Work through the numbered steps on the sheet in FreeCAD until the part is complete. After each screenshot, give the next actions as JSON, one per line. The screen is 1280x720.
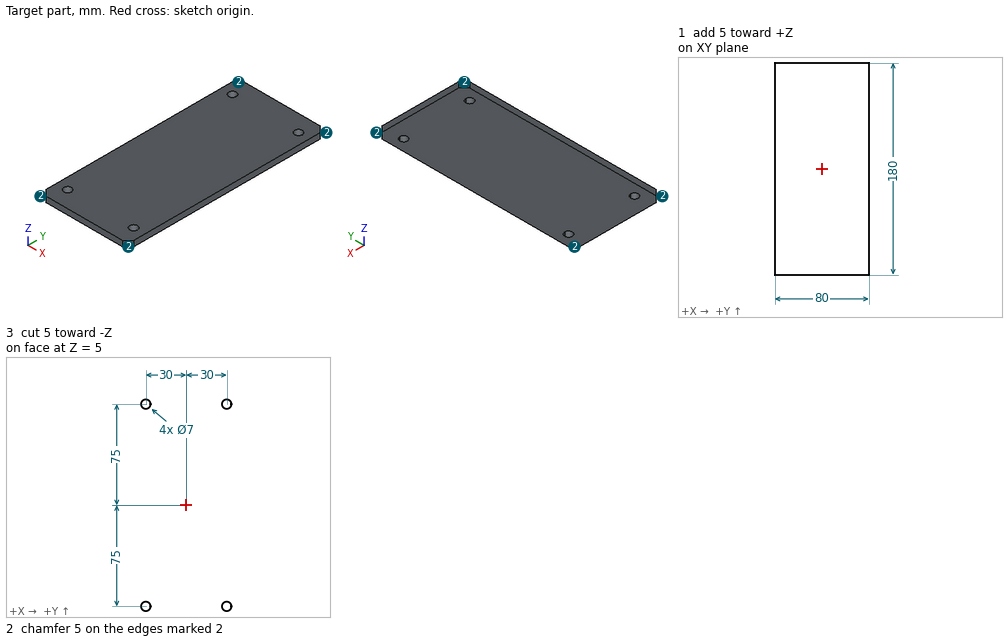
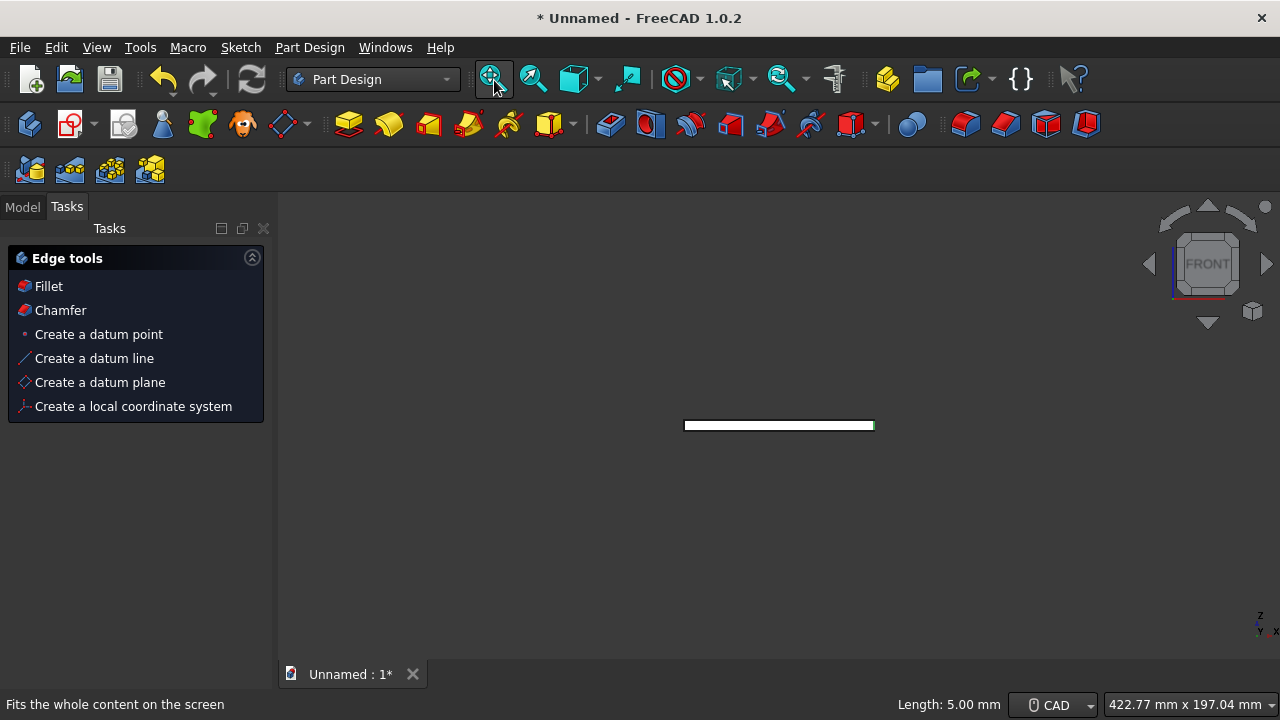
{"action": "scroll", "coordinate": [684, 425], "scroll_direction": "up", "scroll_amount": 7}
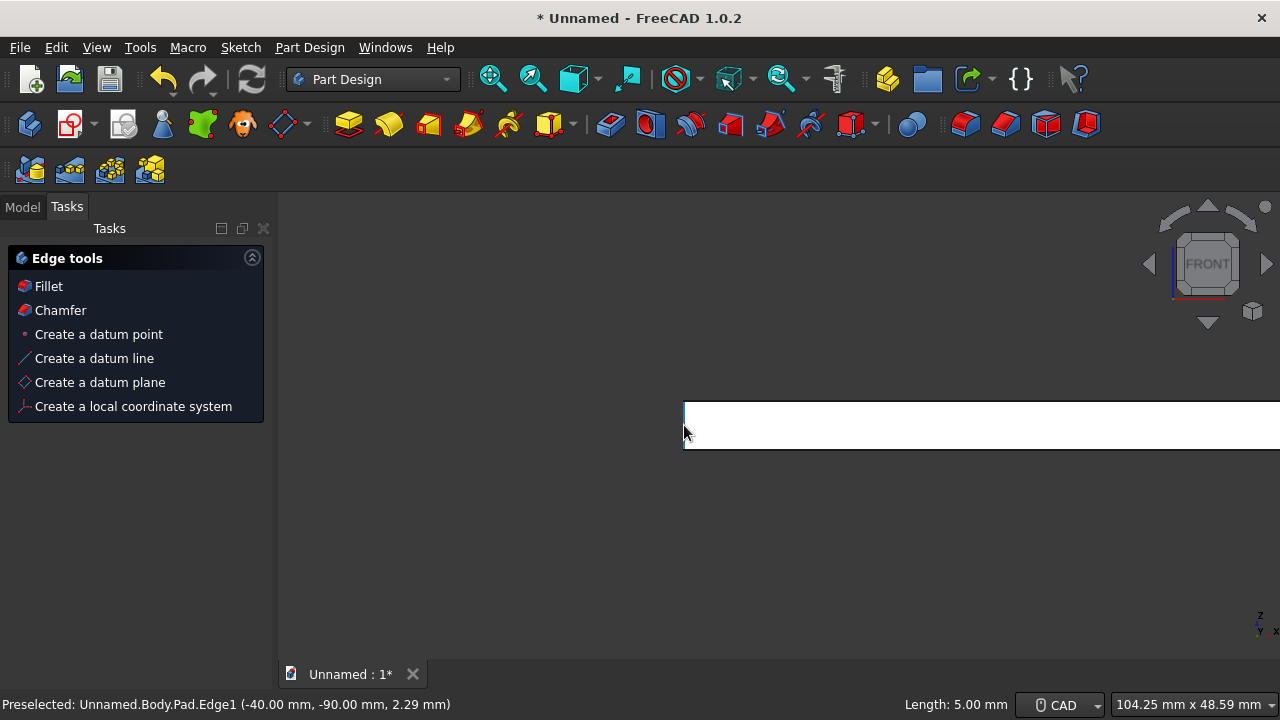
{"action": "left_click", "coordinate": [684, 425], "text": "ctrl"}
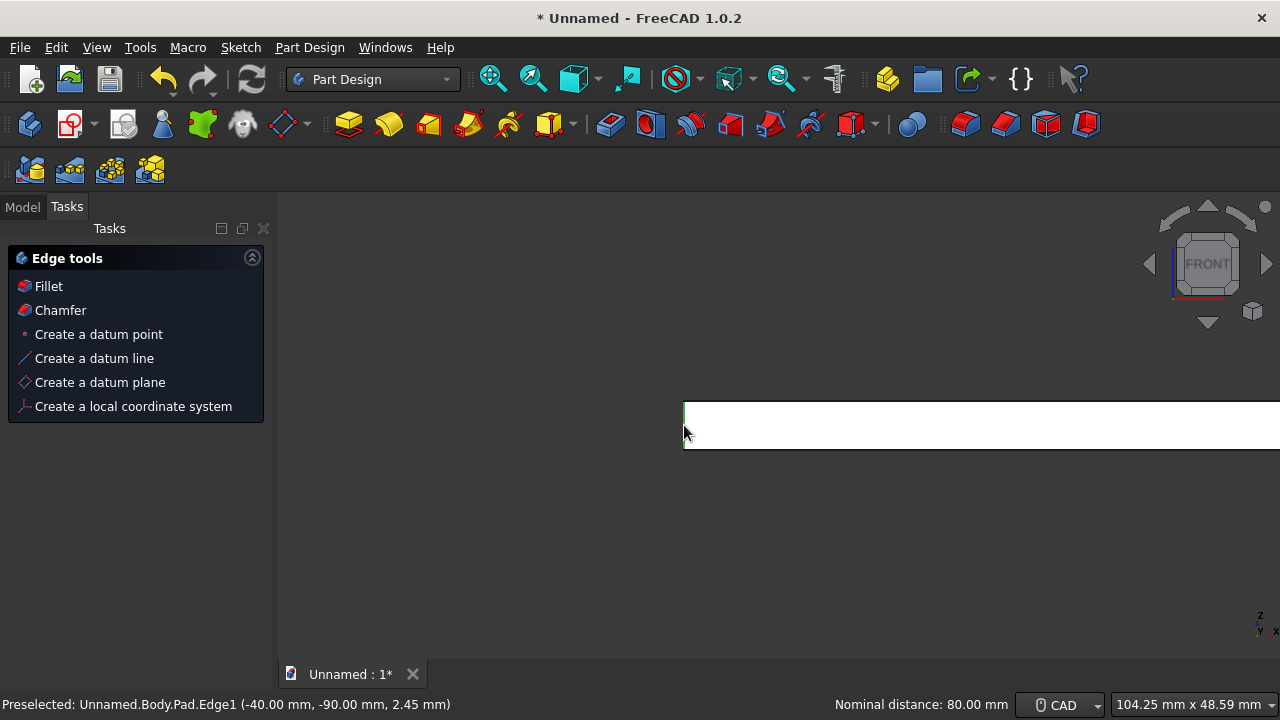
{"action": "left_click", "coordinate": [494, 80]}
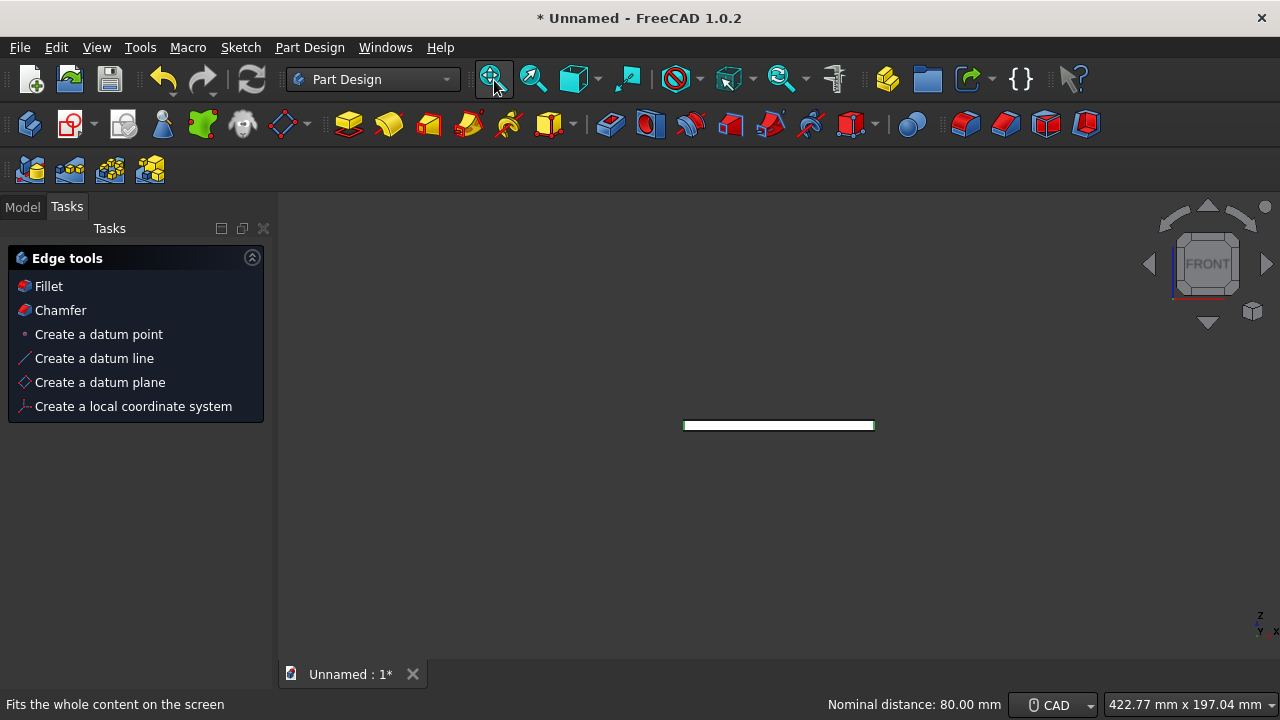
{"action": "key", "text": "3"}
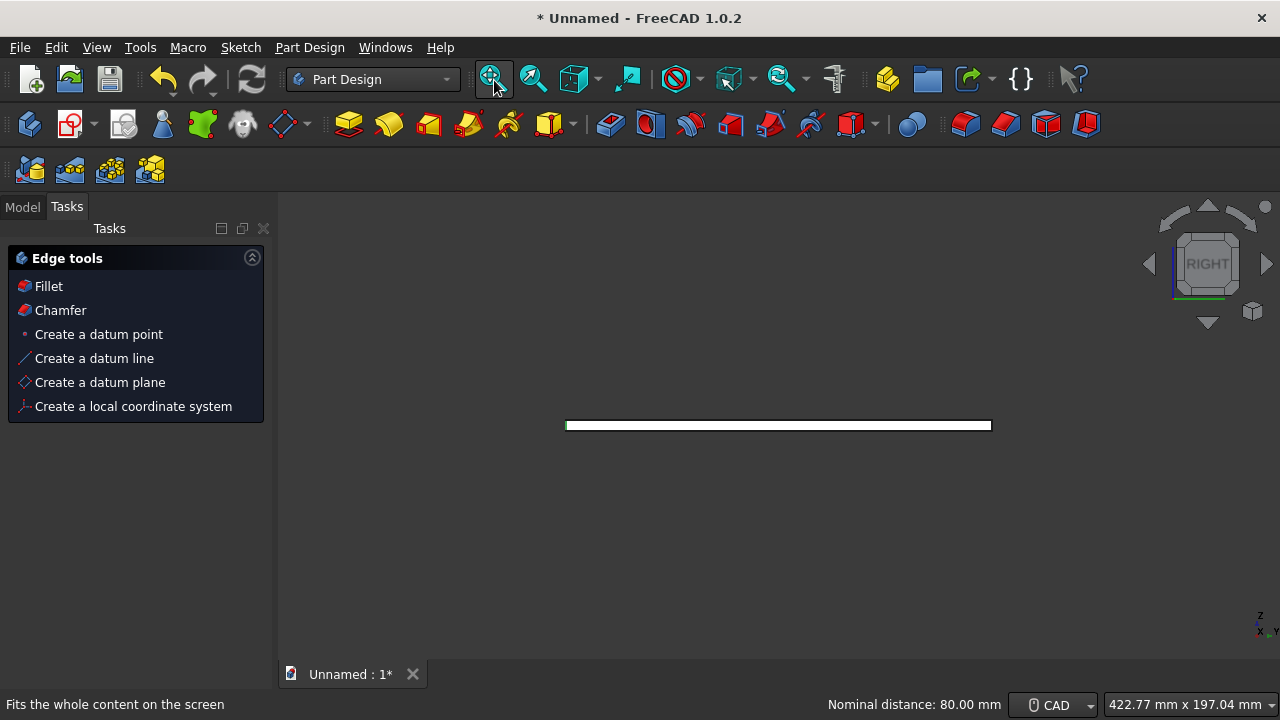
{"action": "left_click", "coordinate": [494, 80]}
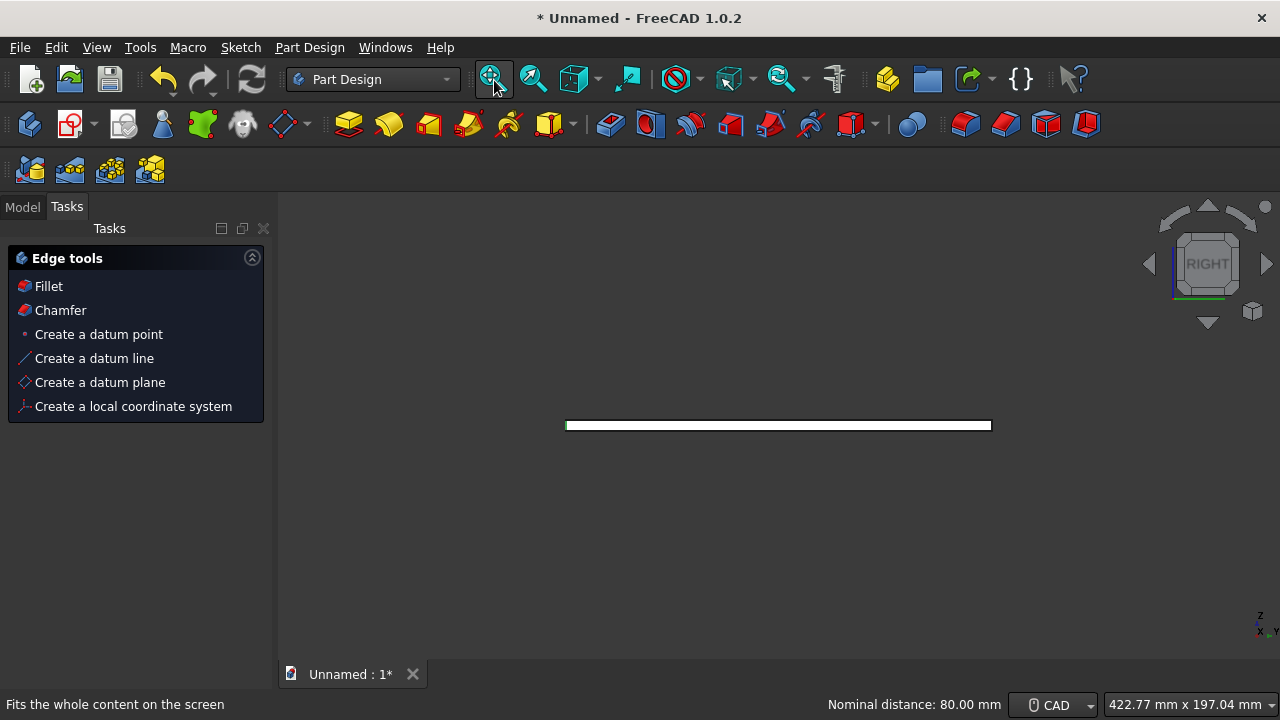
{"action": "scroll", "coordinate": [992, 424], "scroll_direction": "up", "scroll_amount": 7}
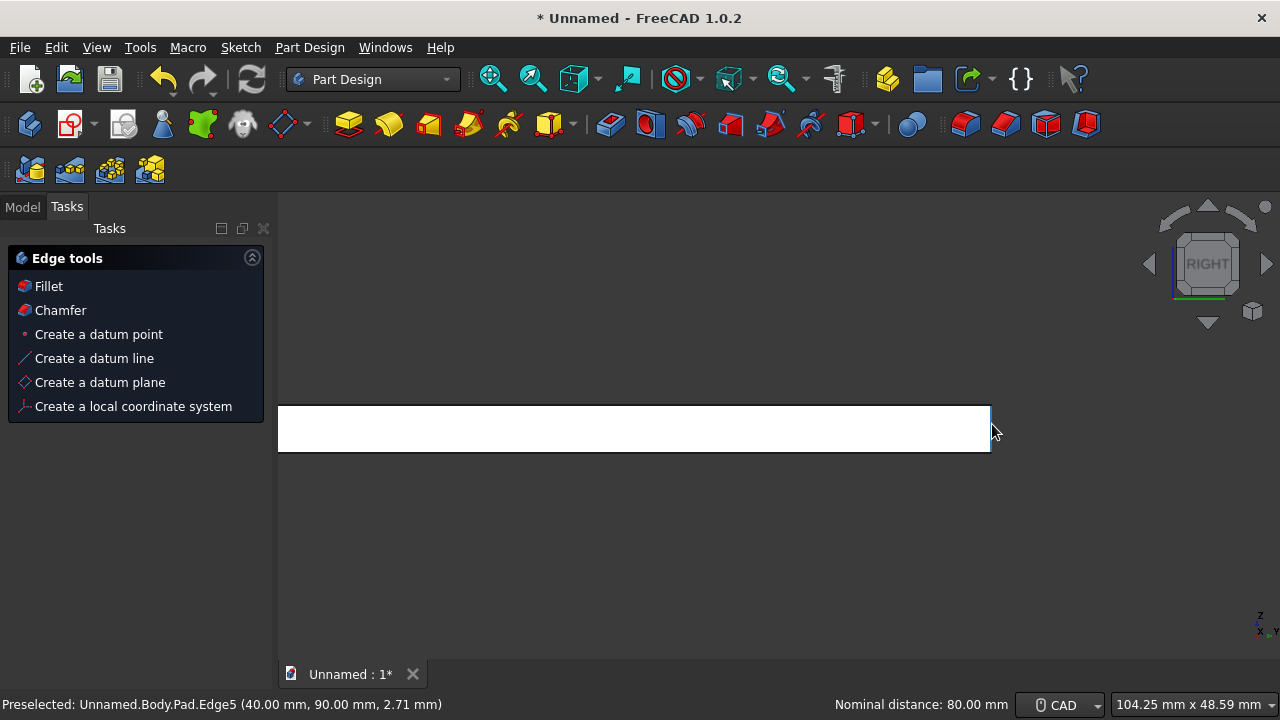
{"action": "left_click", "coordinate": [991, 428], "text": "ctrl"}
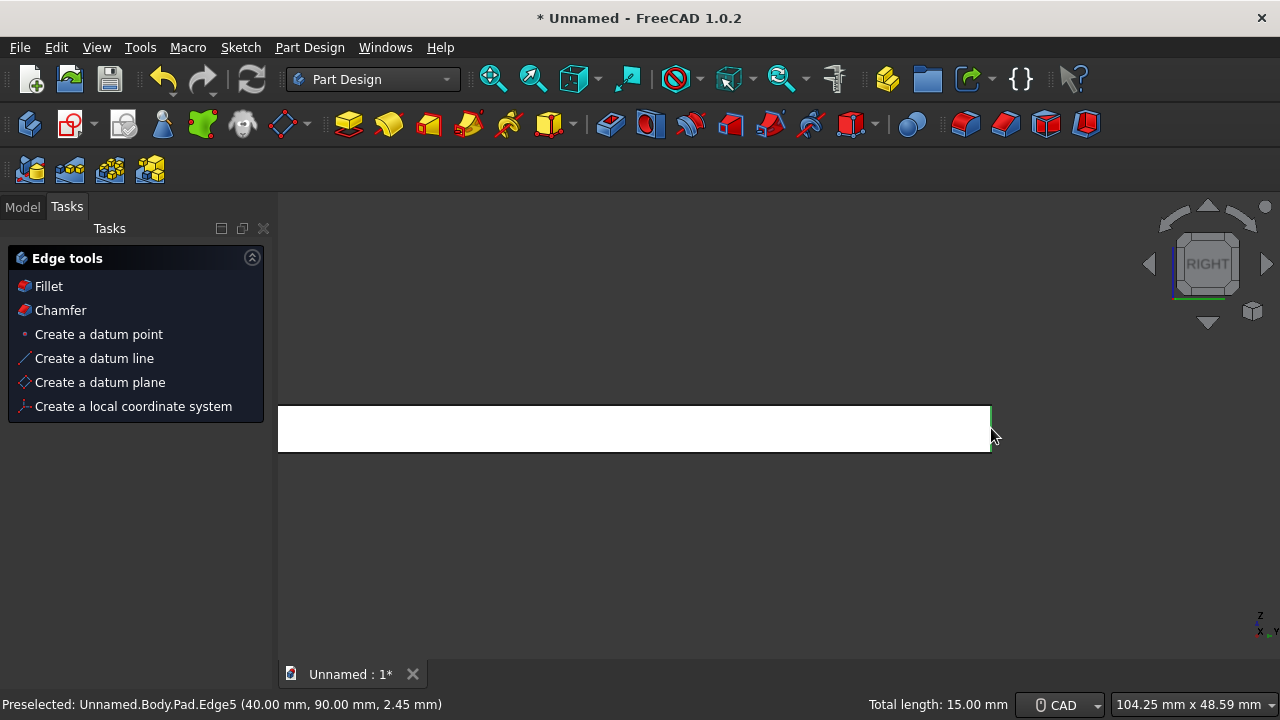
{"action": "left_click", "coordinate": [494, 80]}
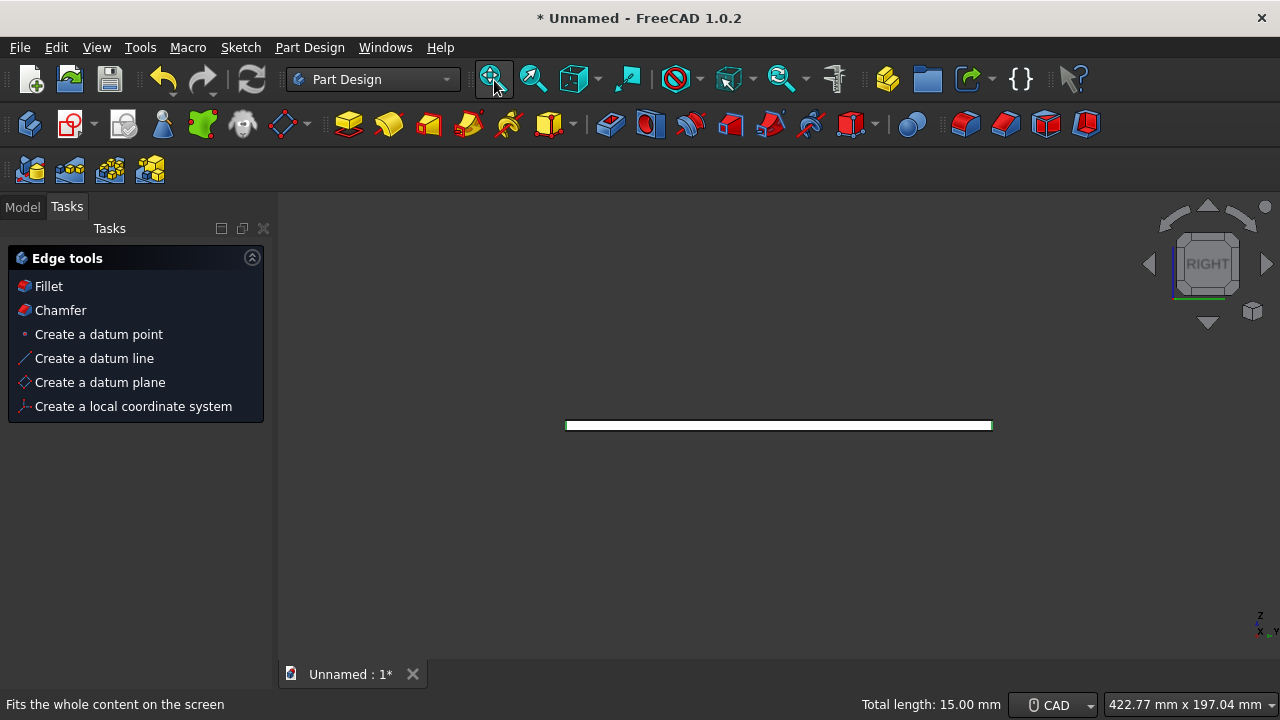
{"action": "key", "text": "5"}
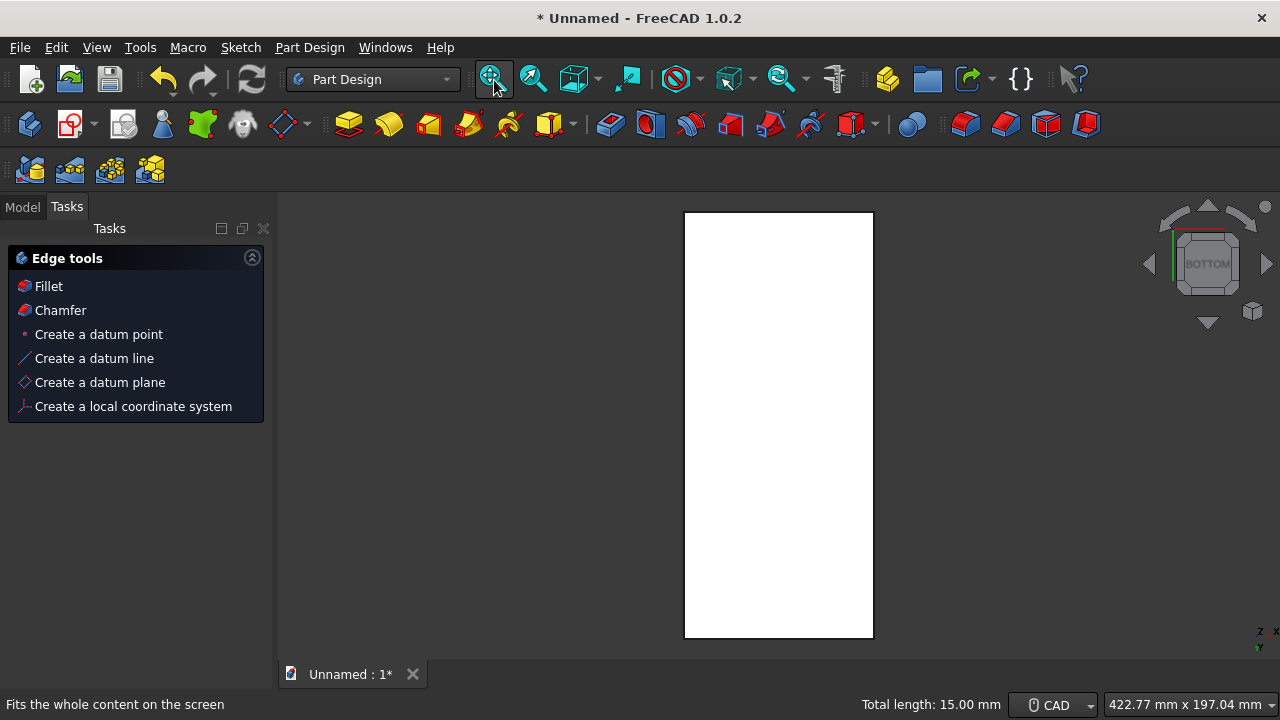
{"action": "key", "text": "4"}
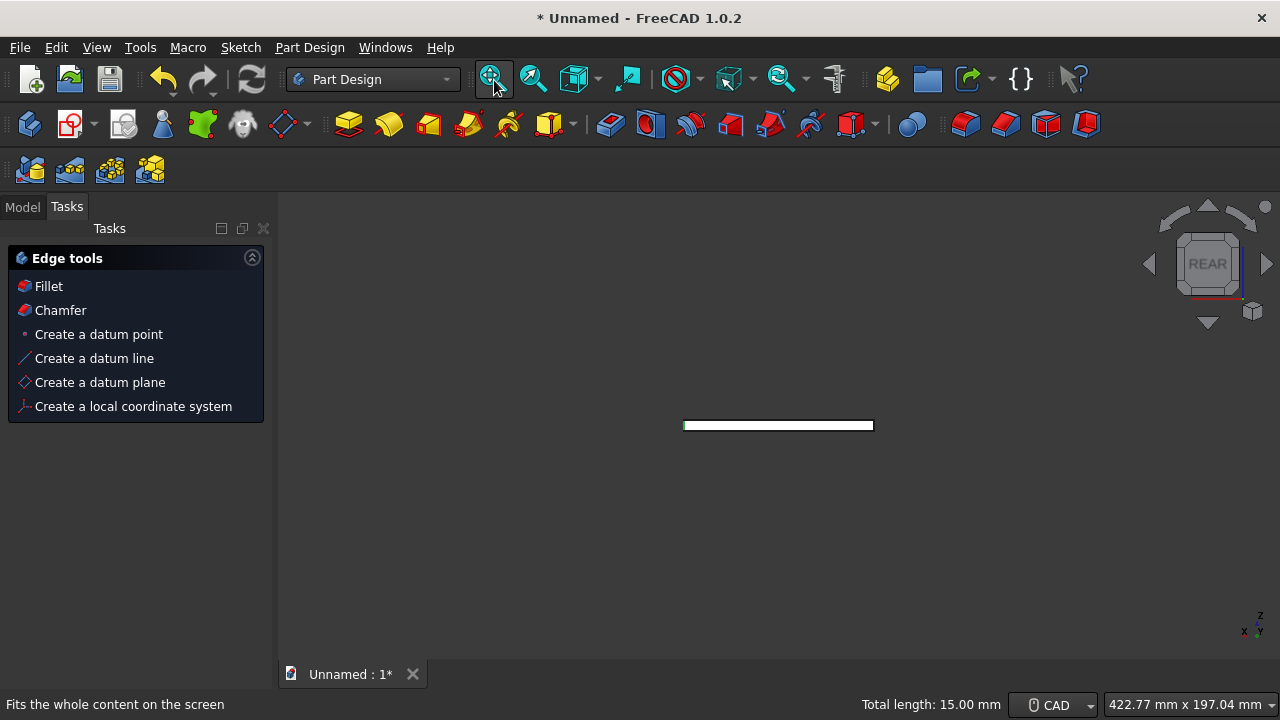
{"action": "left_click", "coordinate": [494, 80]}